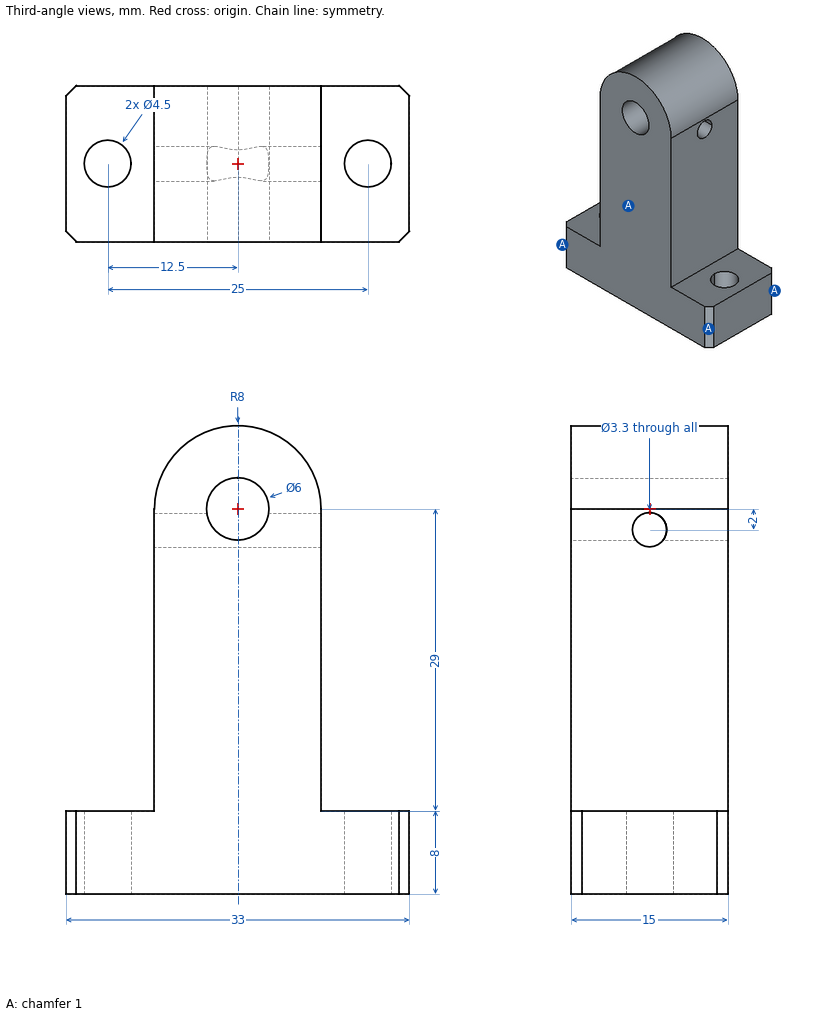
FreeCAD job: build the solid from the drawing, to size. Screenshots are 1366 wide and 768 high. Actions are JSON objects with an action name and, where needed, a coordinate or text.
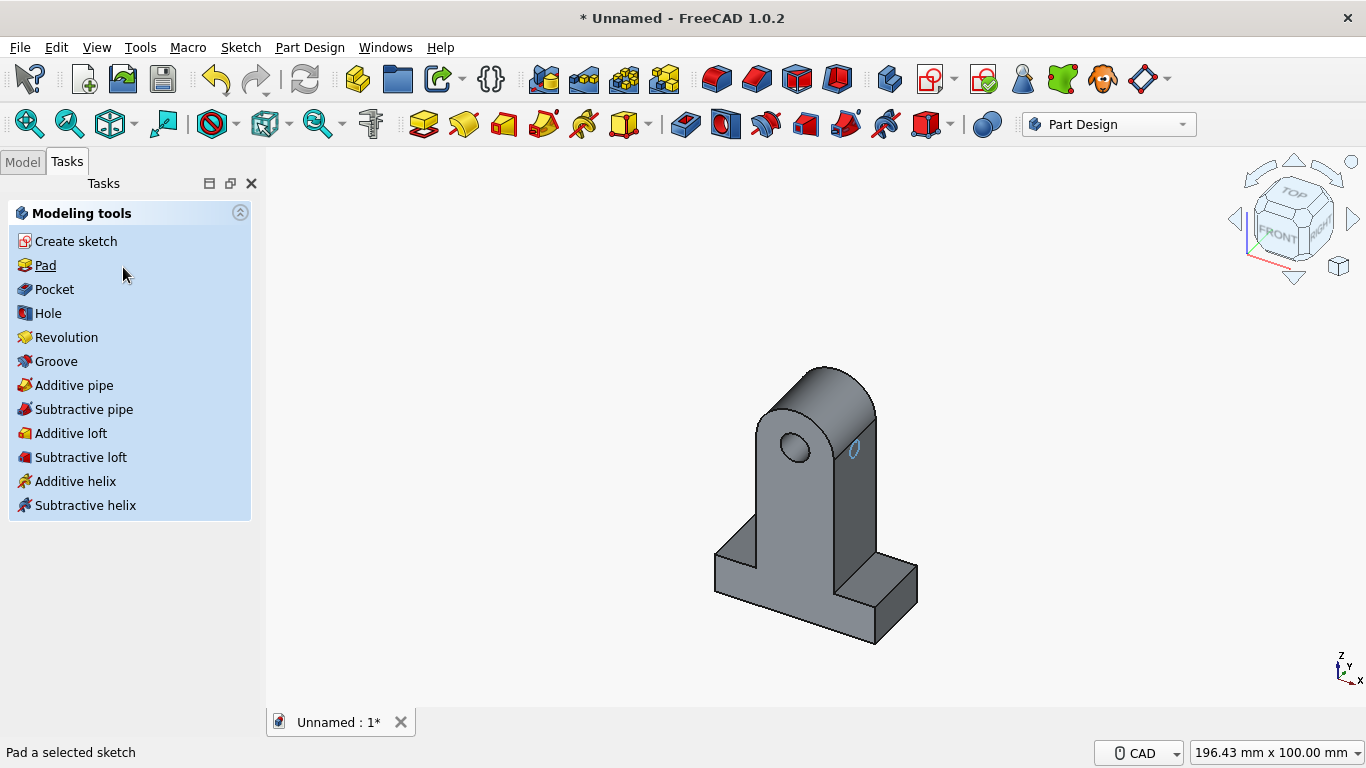
{"action": "left_click", "coordinate": [726, 124]}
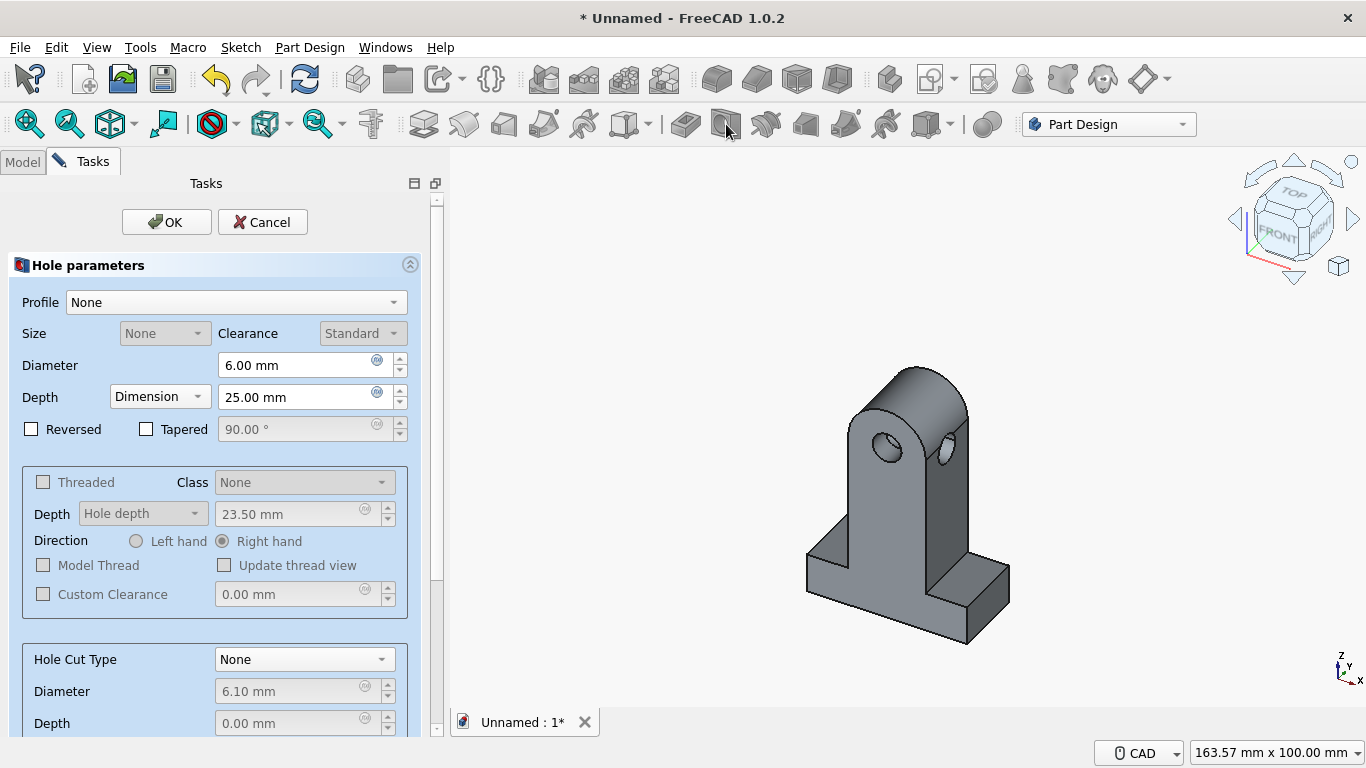
{"action": "triple_click", "coordinate": [305, 365]}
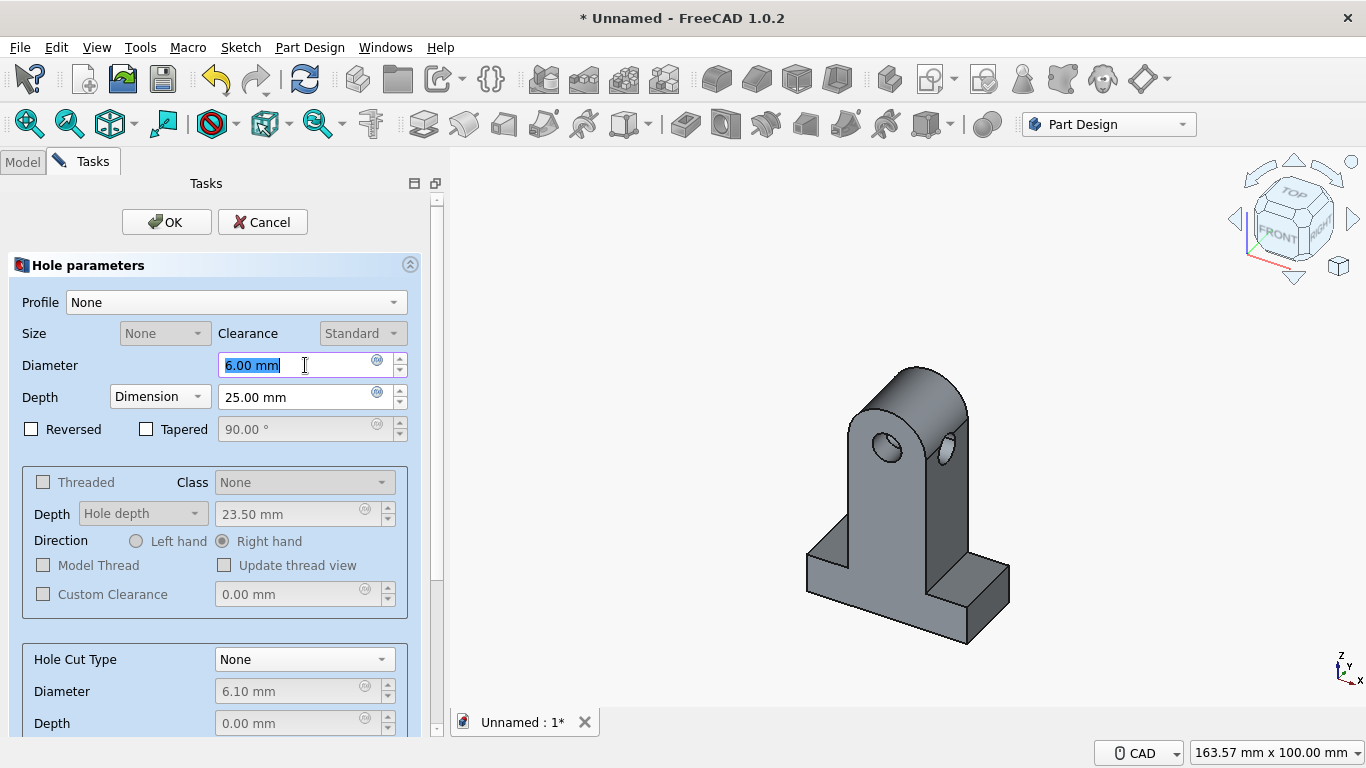
{"action": "type", "text": "3.3"}
{"action": "key", "text": "Tab"}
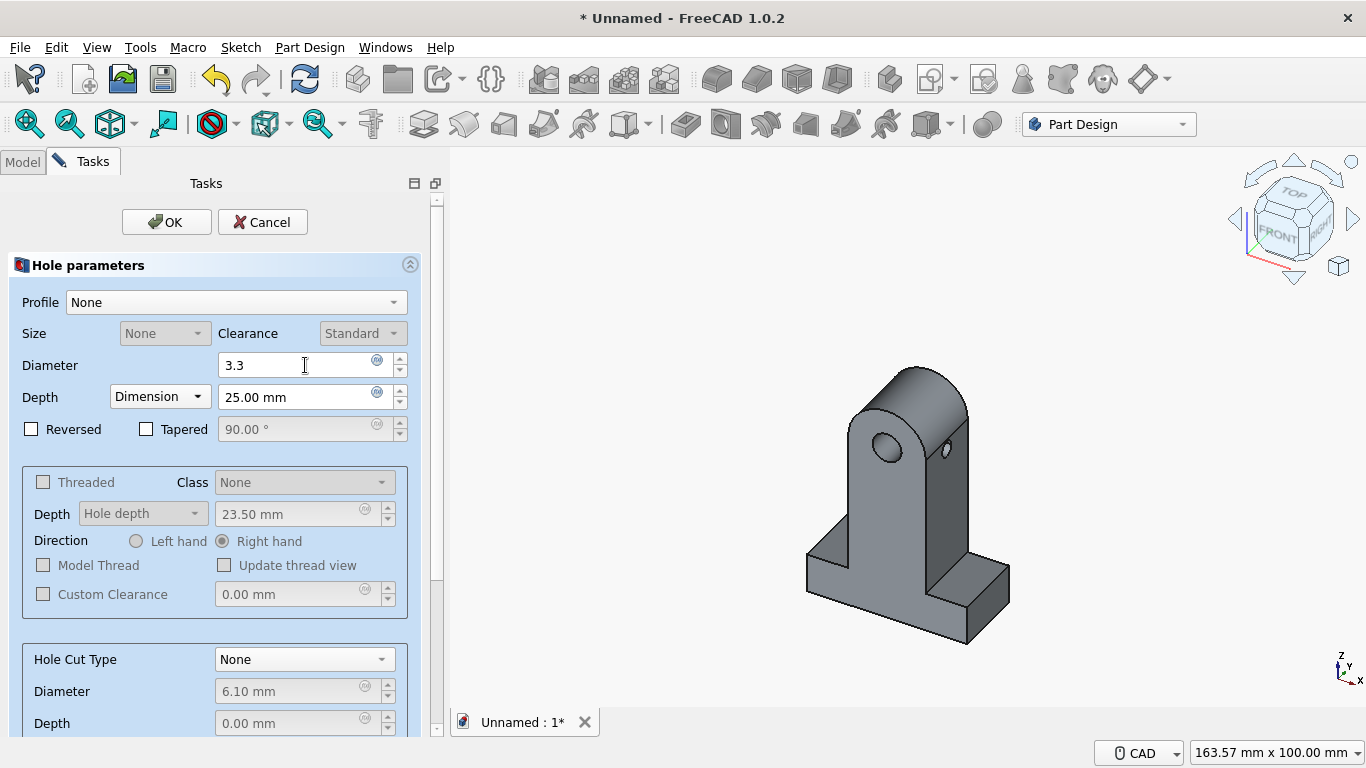
{"action": "left_click", "coordinate": [161, 396]}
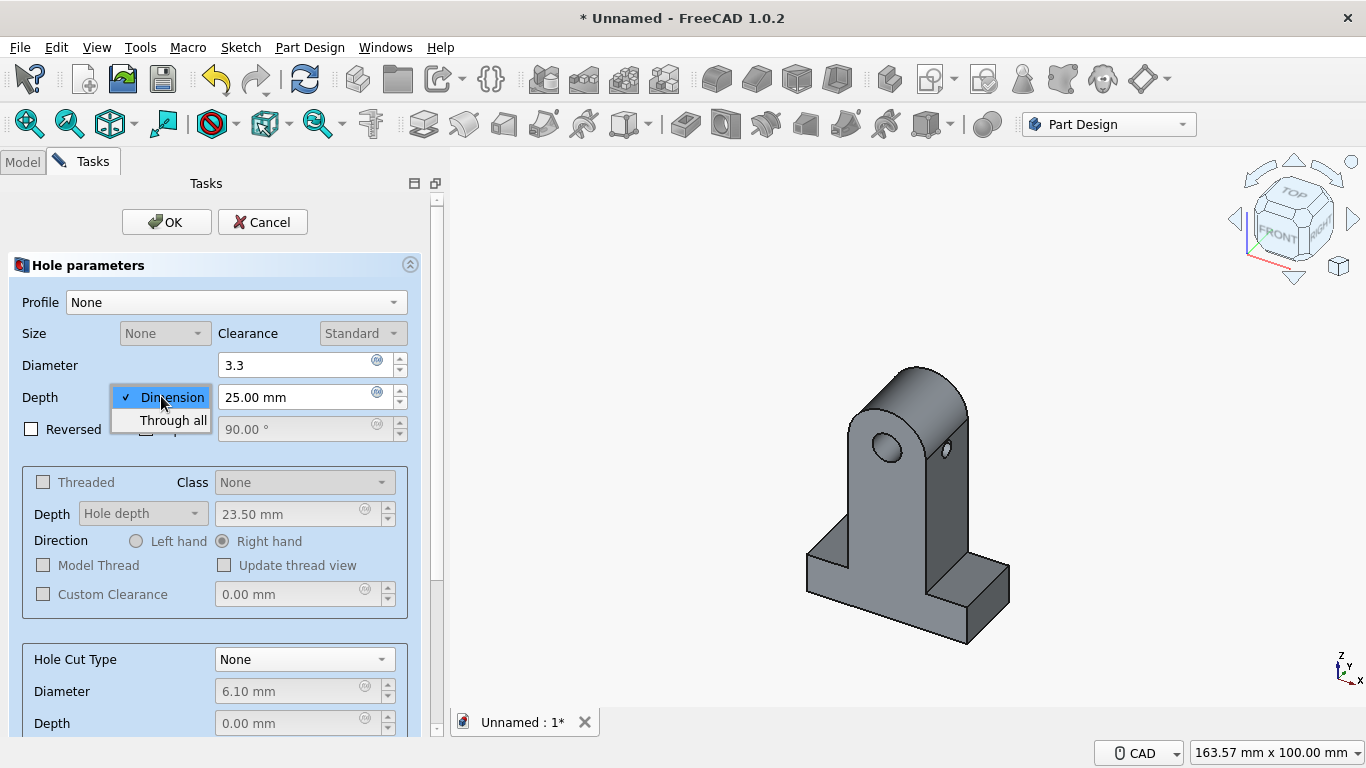
{"action": "left_click", "coordinate": [160, 420]}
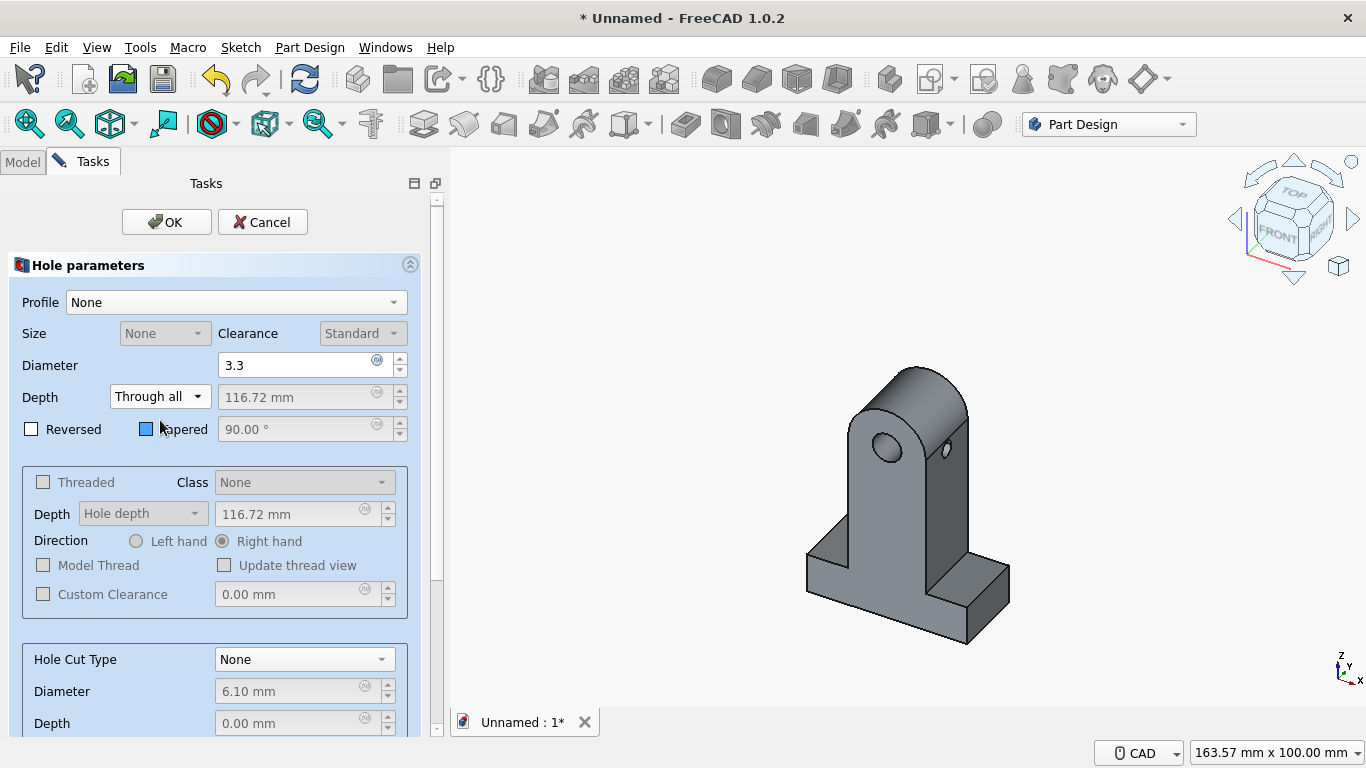
{"action": "left_click", "coordinate": [167, 222]}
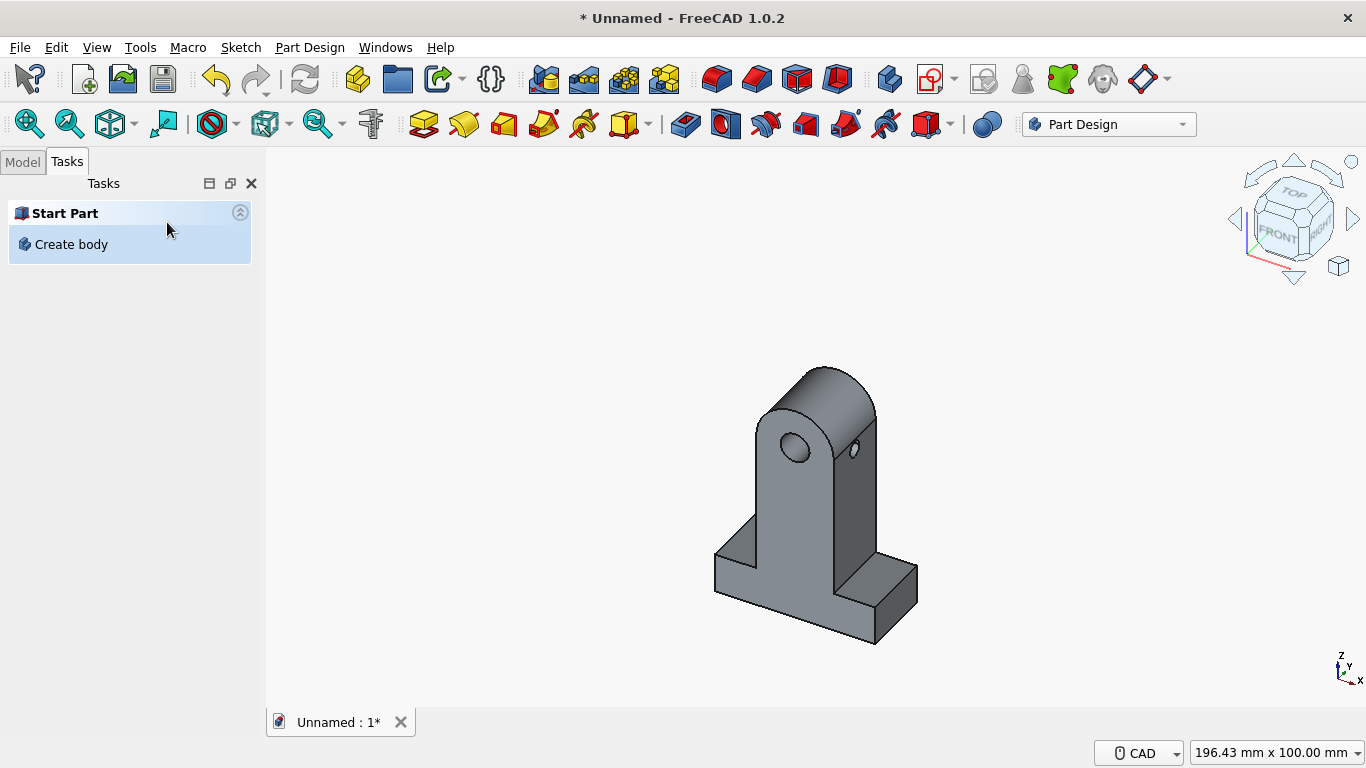
{"action": "left_click", "coordinate": [881, 573]}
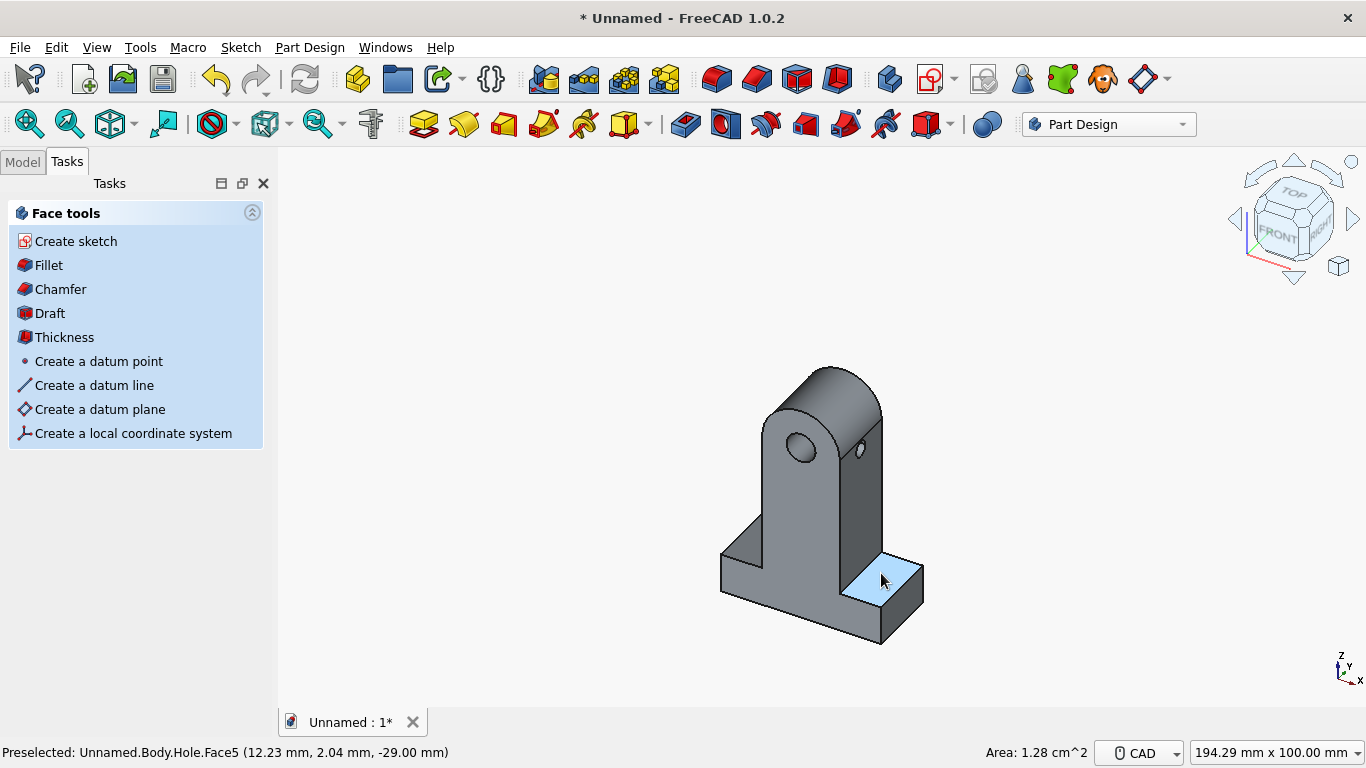
{"action": "left_click", "coordinate": [930, 80]}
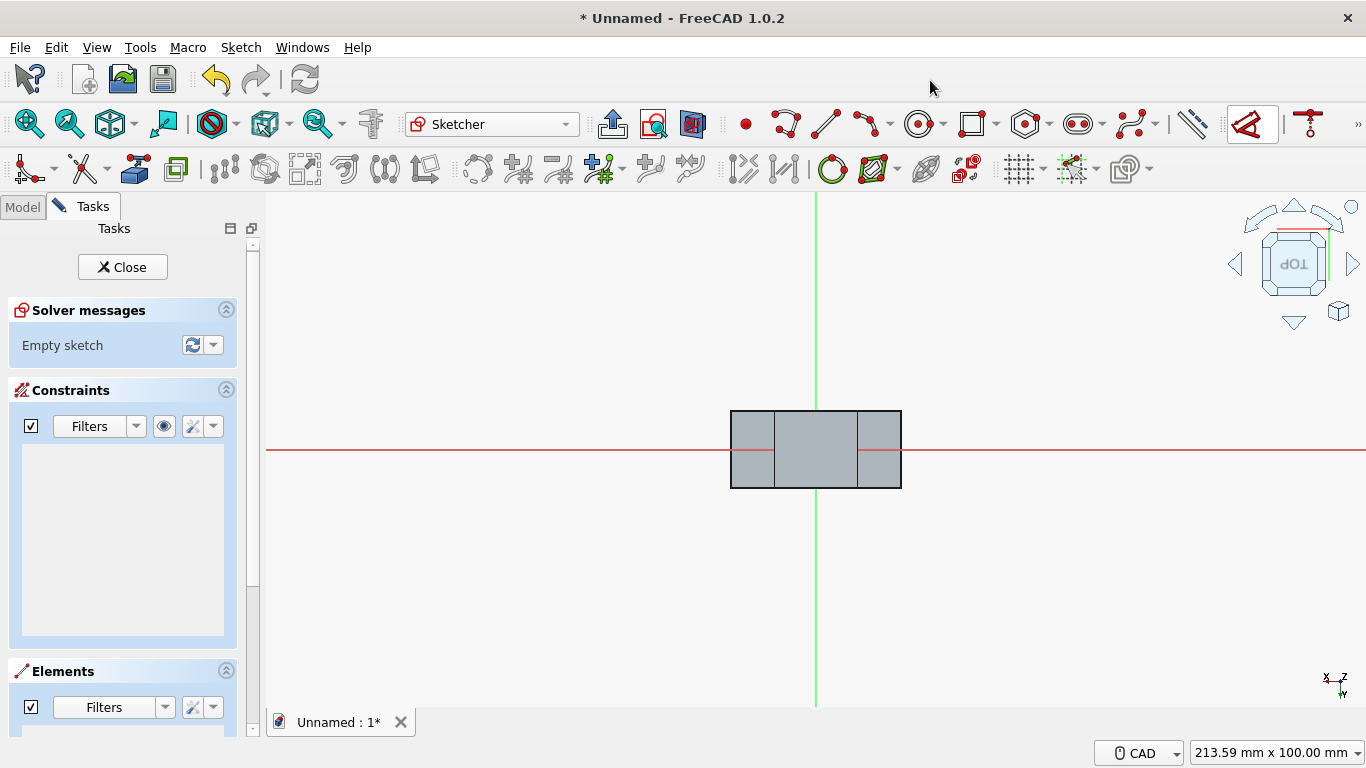
{"action": "left_click", "coordinate": [694, 124]}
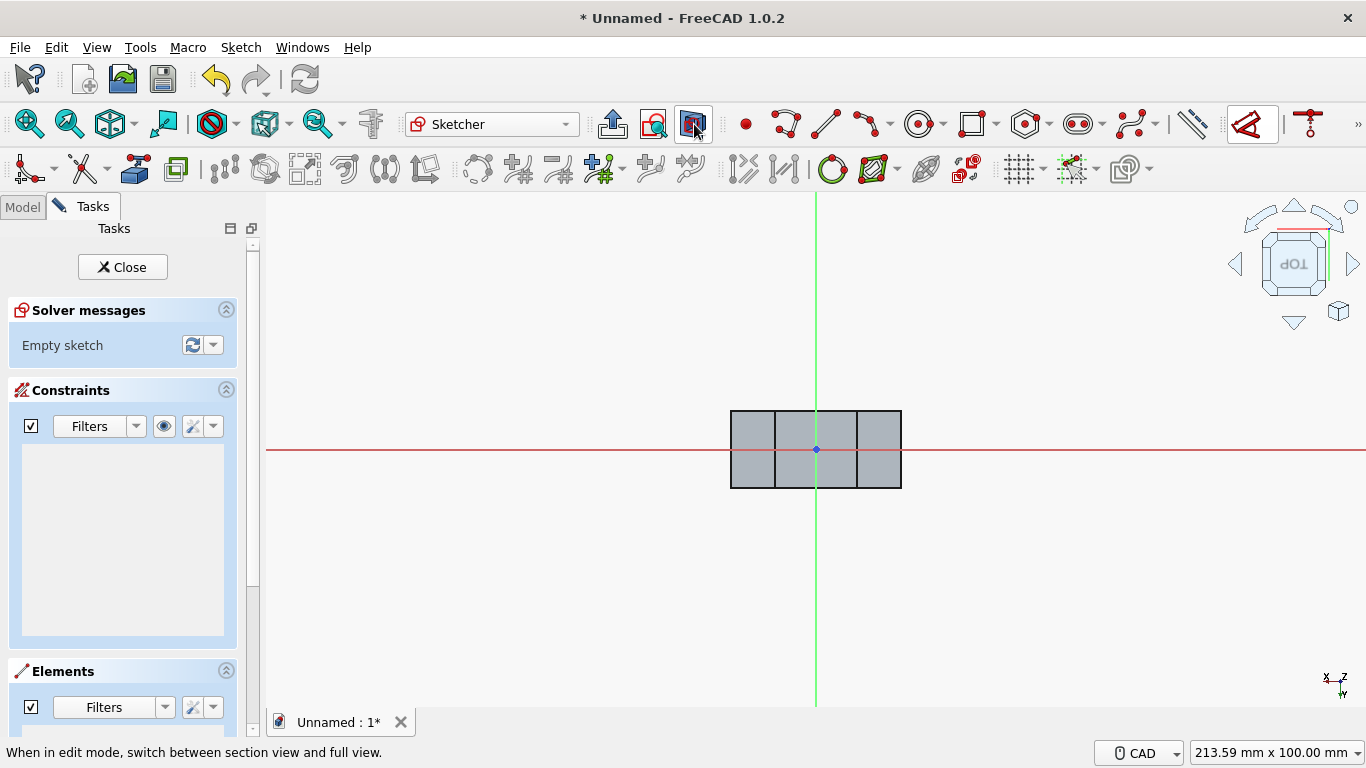
{"action": "scroll", "coordinate": [838, 449], "scroll_direction": "up", "scroll_amount": 7}